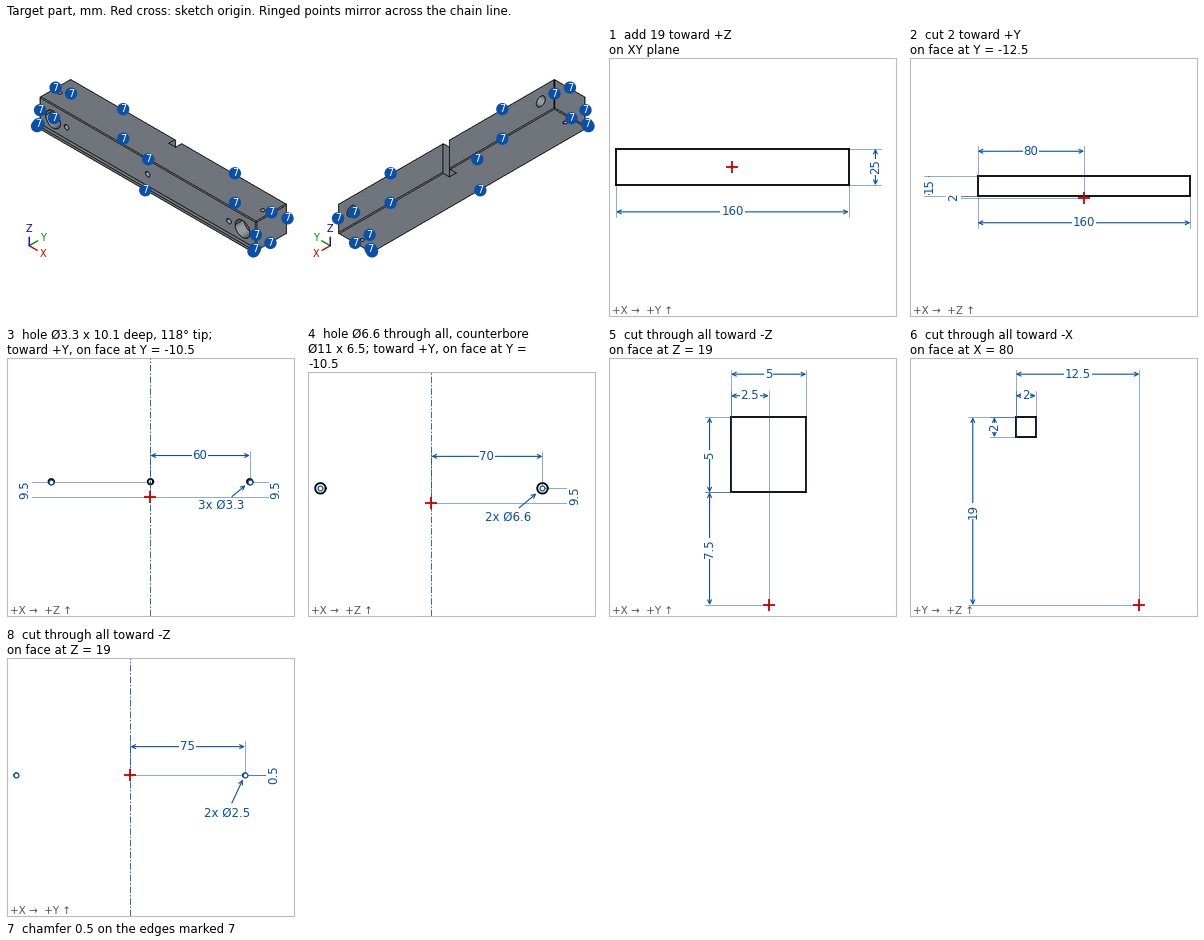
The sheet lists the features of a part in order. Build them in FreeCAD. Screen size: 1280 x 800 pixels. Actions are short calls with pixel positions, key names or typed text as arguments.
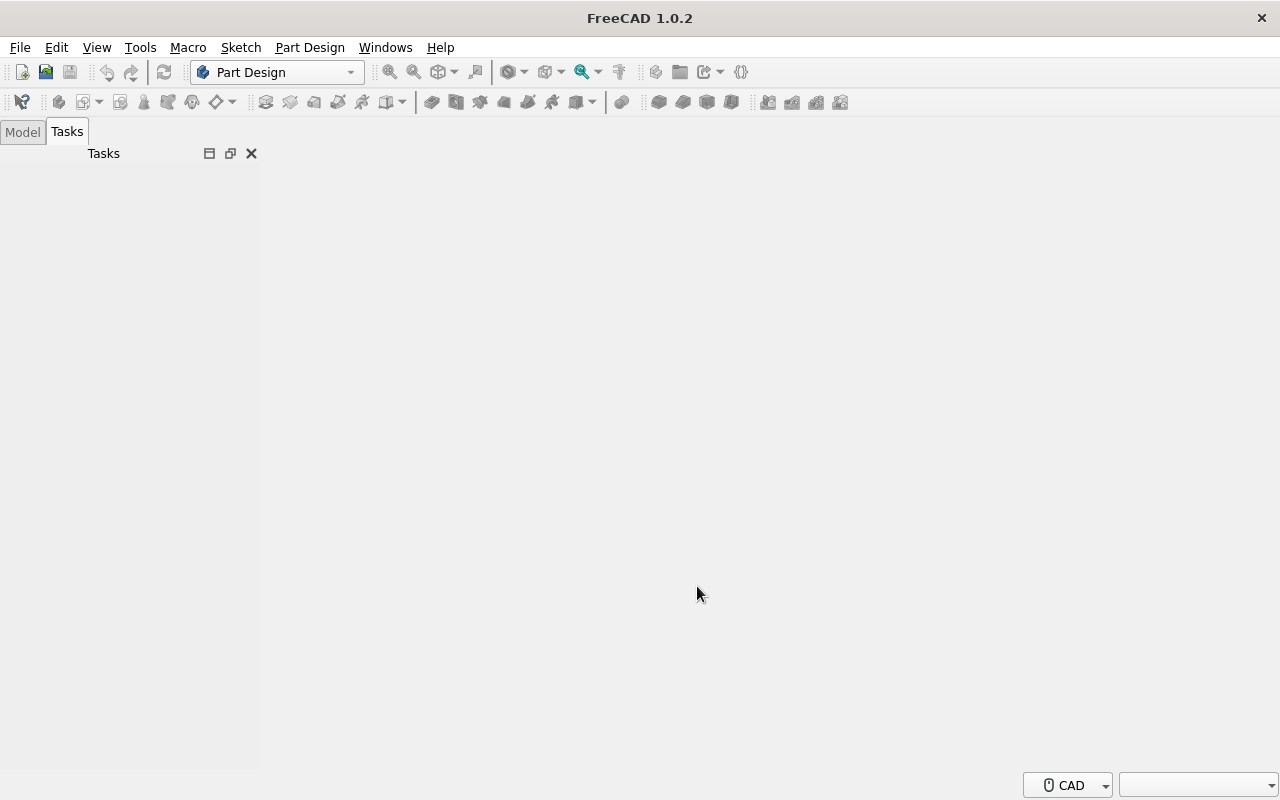
click(22, 72)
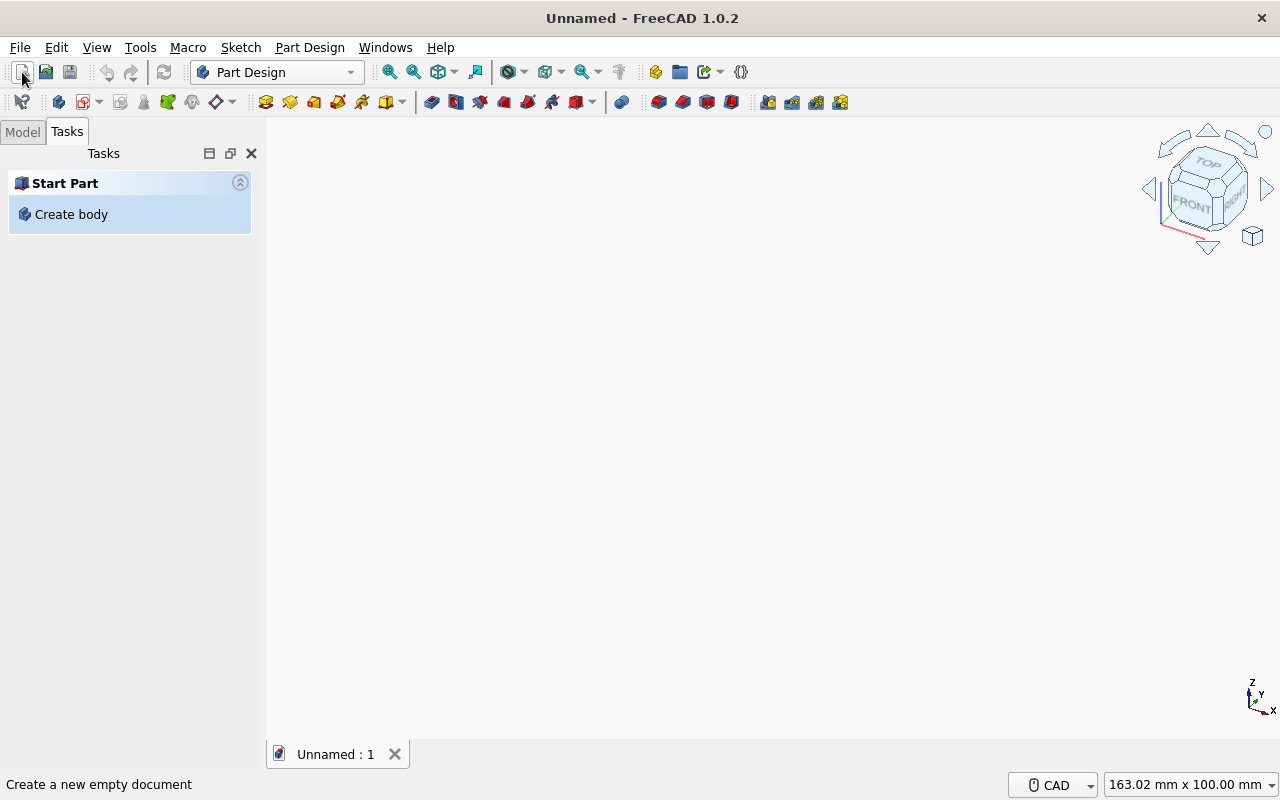
click(84, 102)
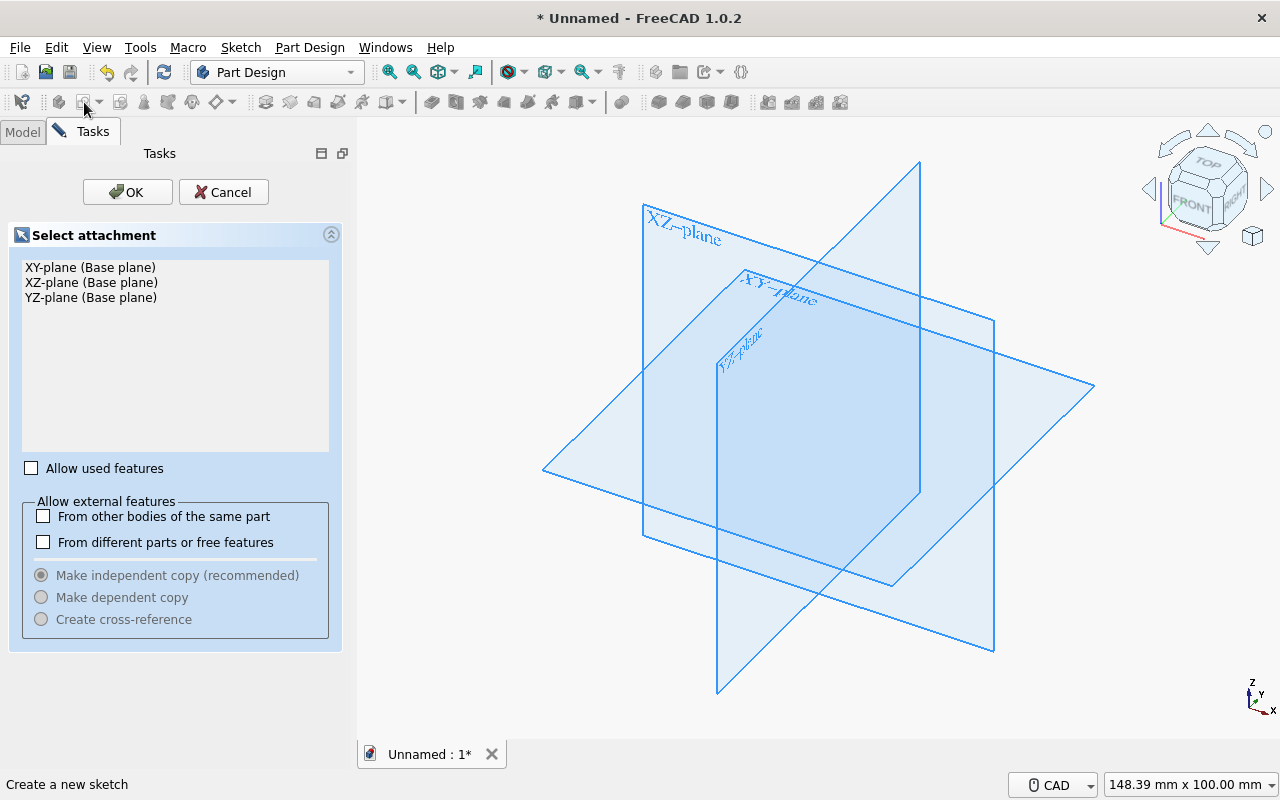
click(82, 268)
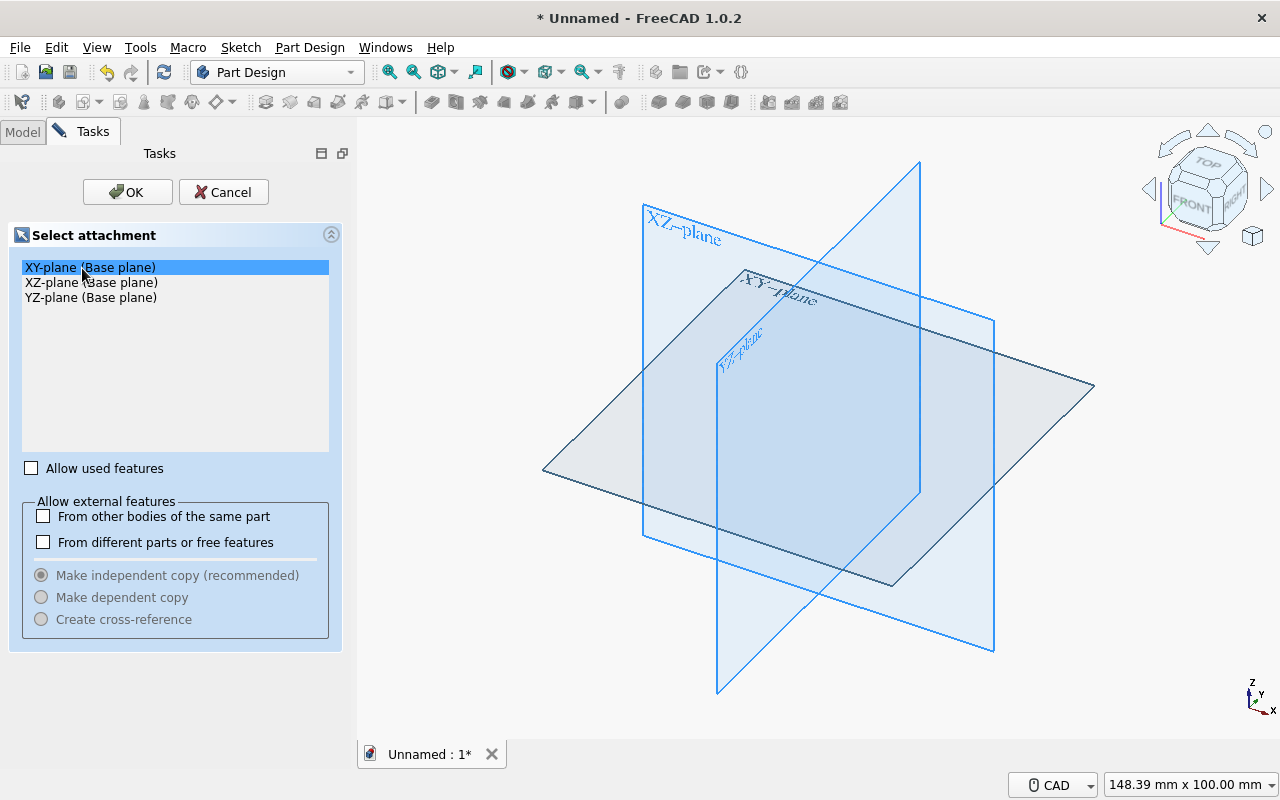
click(128, 192)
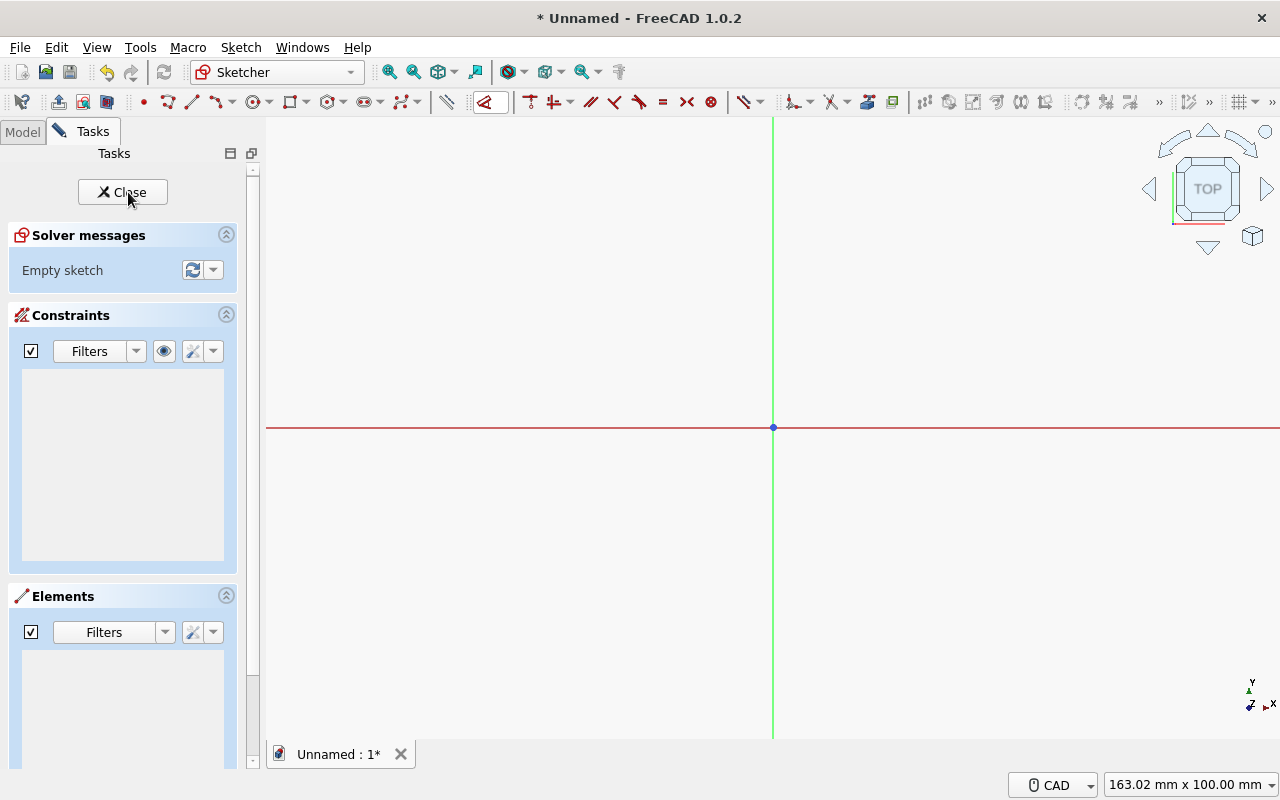
scroll(621, 428, down, 3)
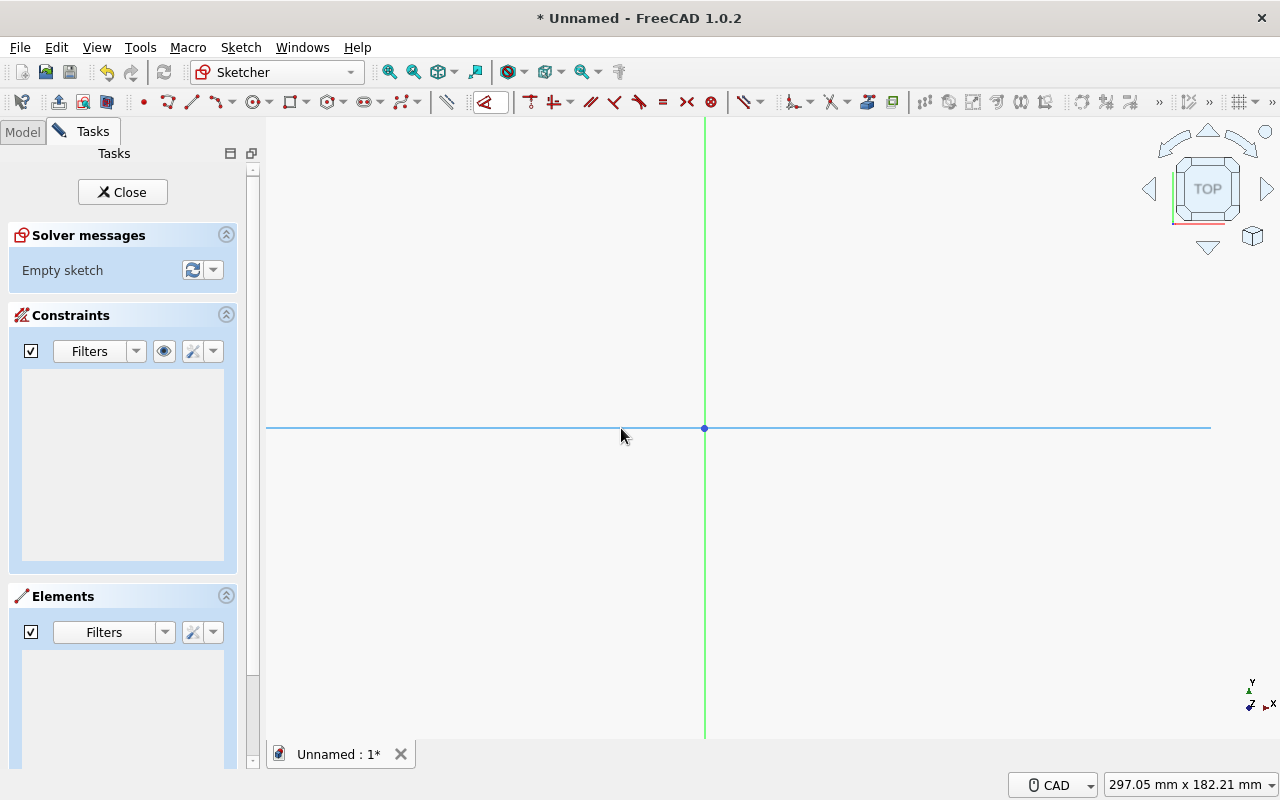
key(g)
key(v)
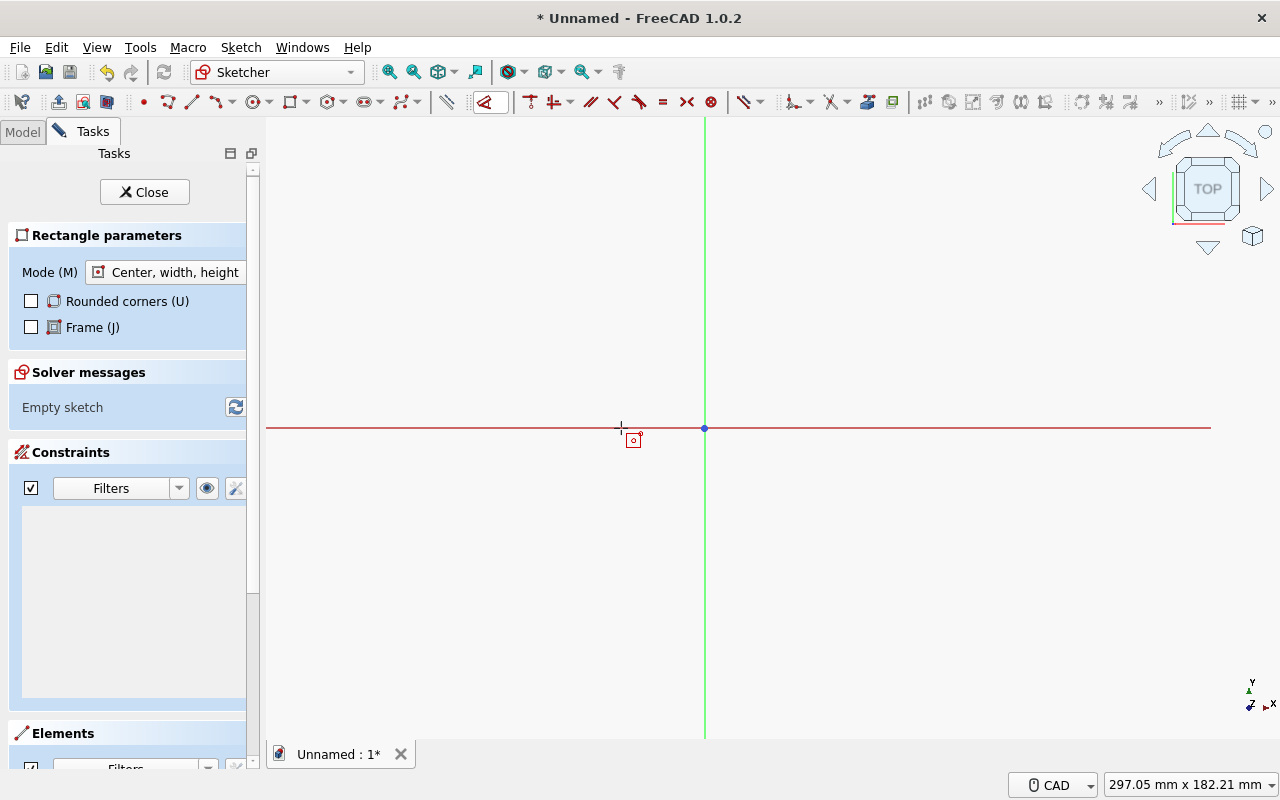
click(705, 428)
click(978, 386)
key(Escape)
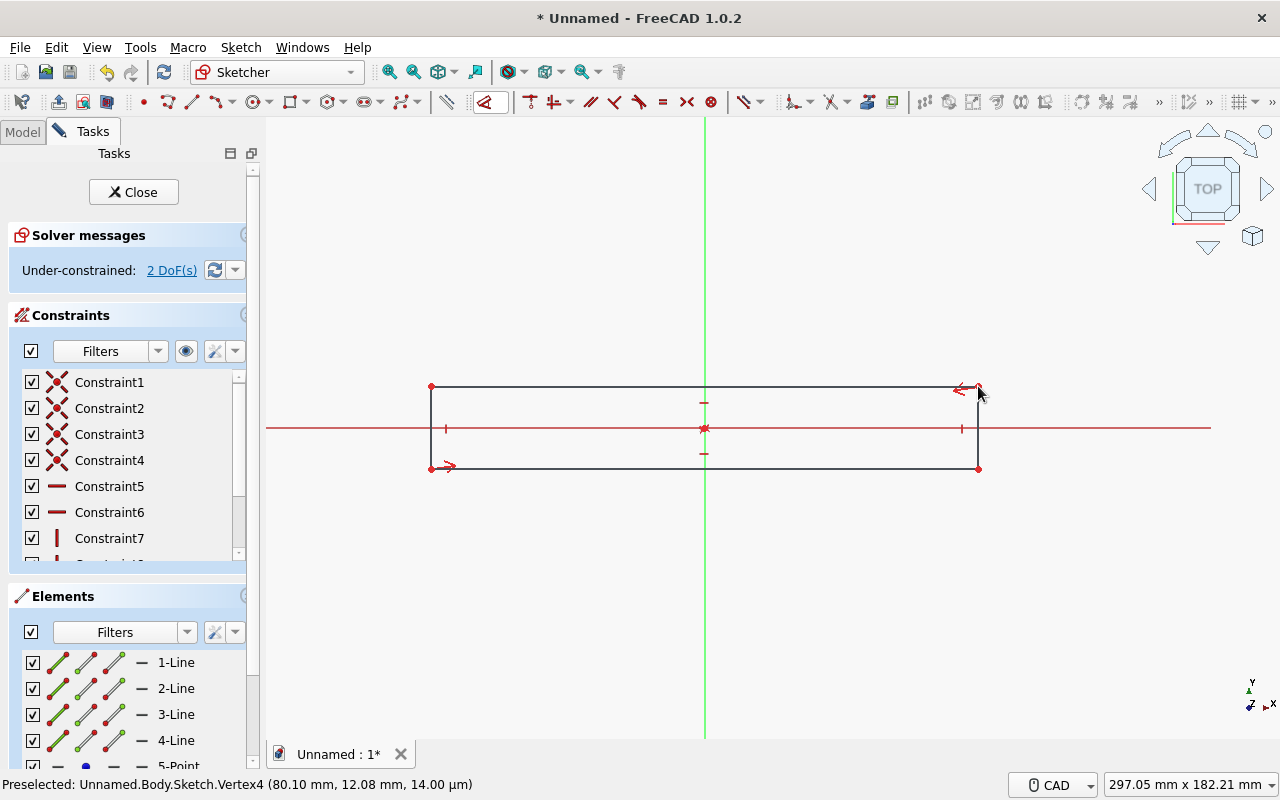
click(484, 102)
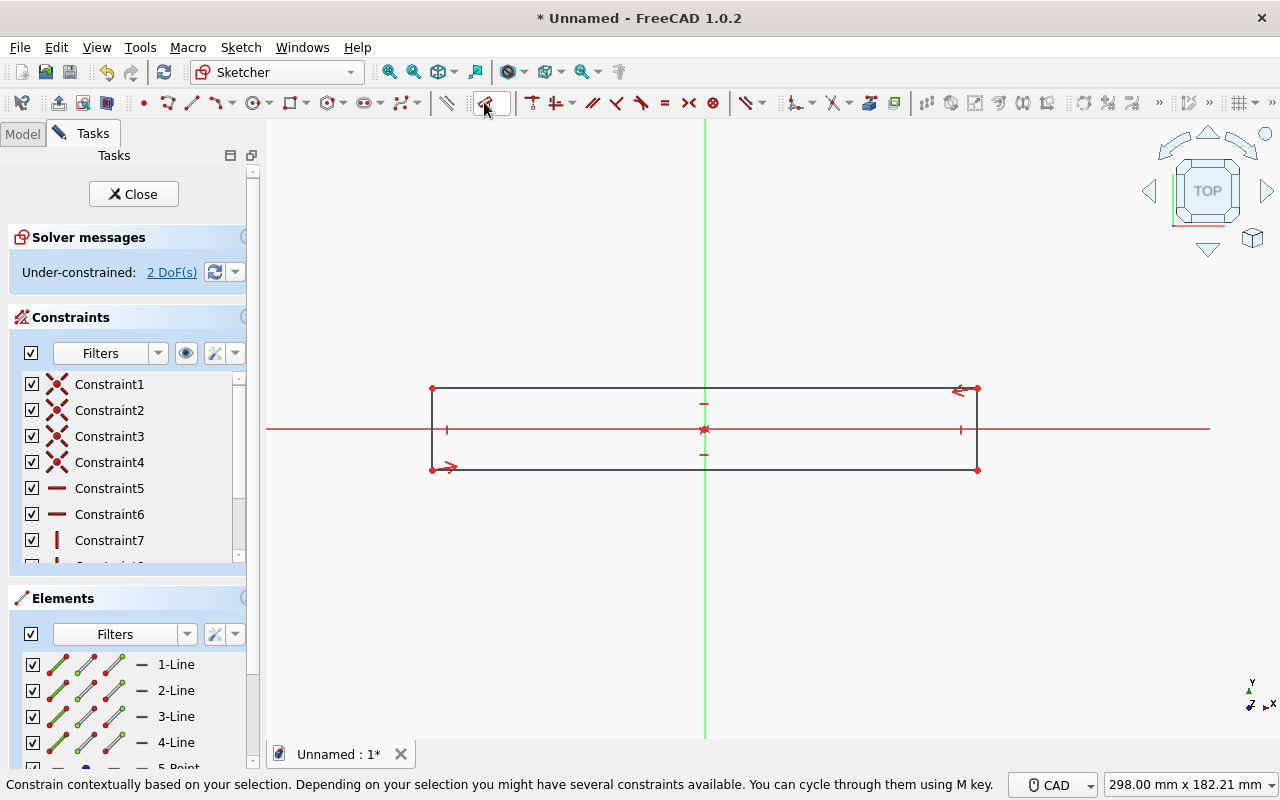
click(977, 446)
click(1011, 410)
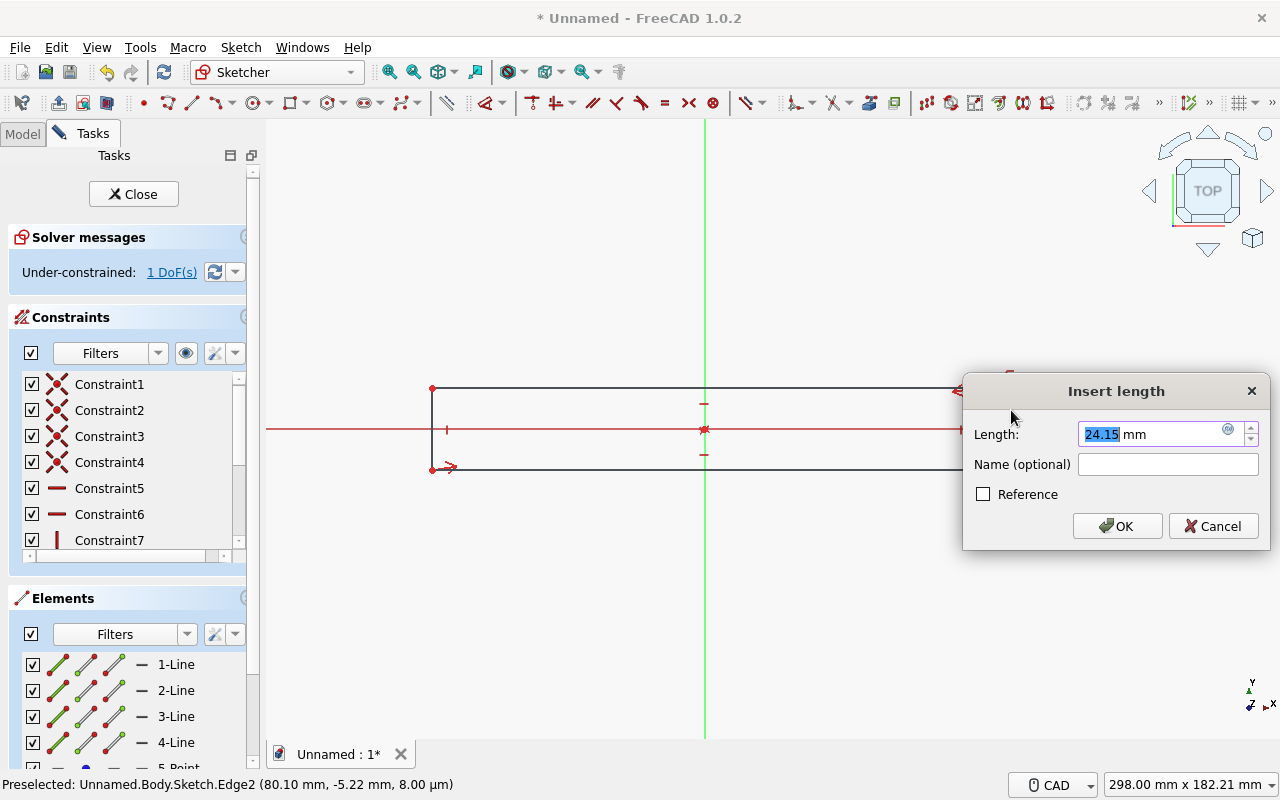
text(25)
key(Return)